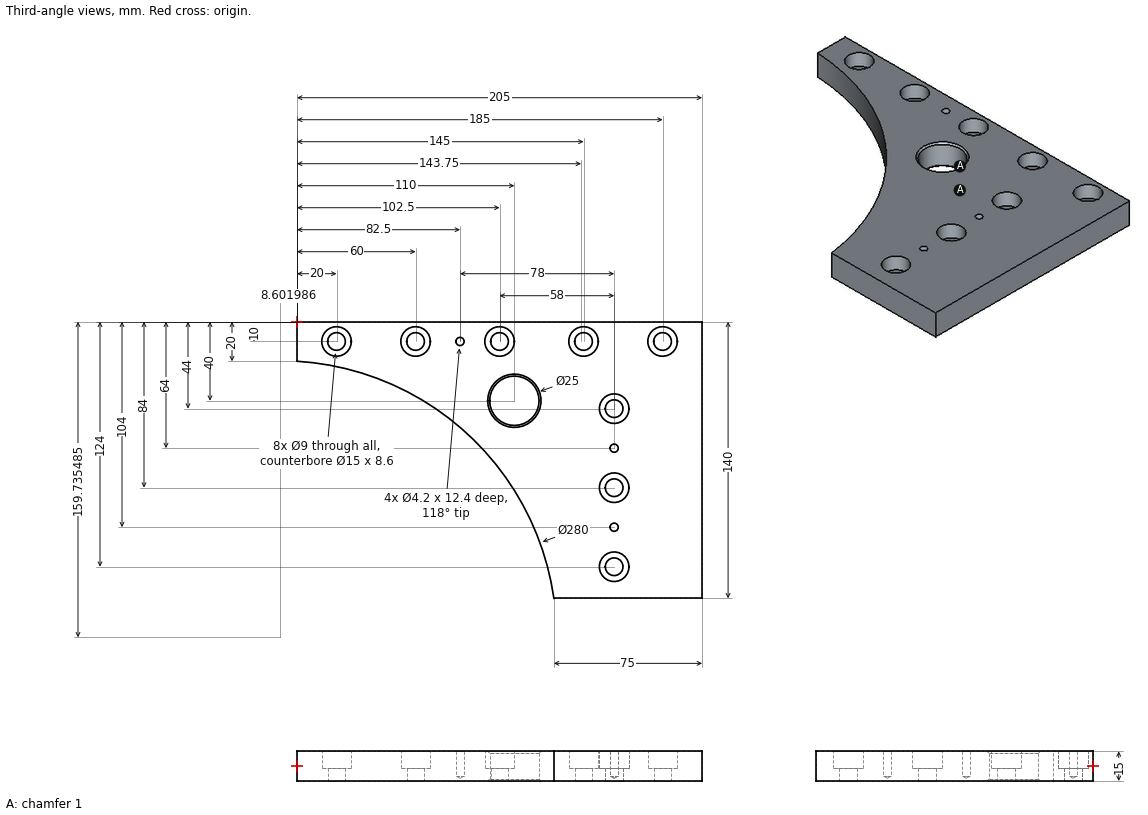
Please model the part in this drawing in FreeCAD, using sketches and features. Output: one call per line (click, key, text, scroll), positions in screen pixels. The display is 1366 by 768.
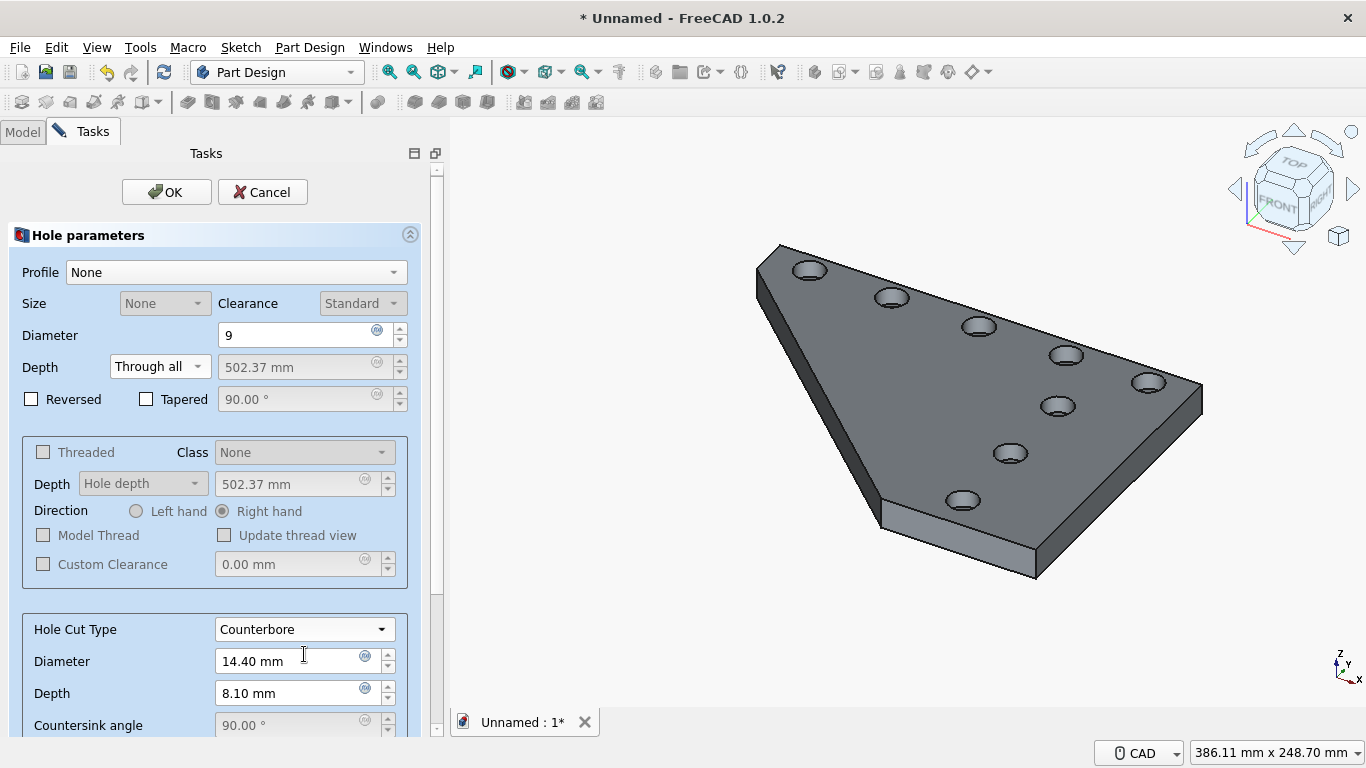
triple_click(298, 661)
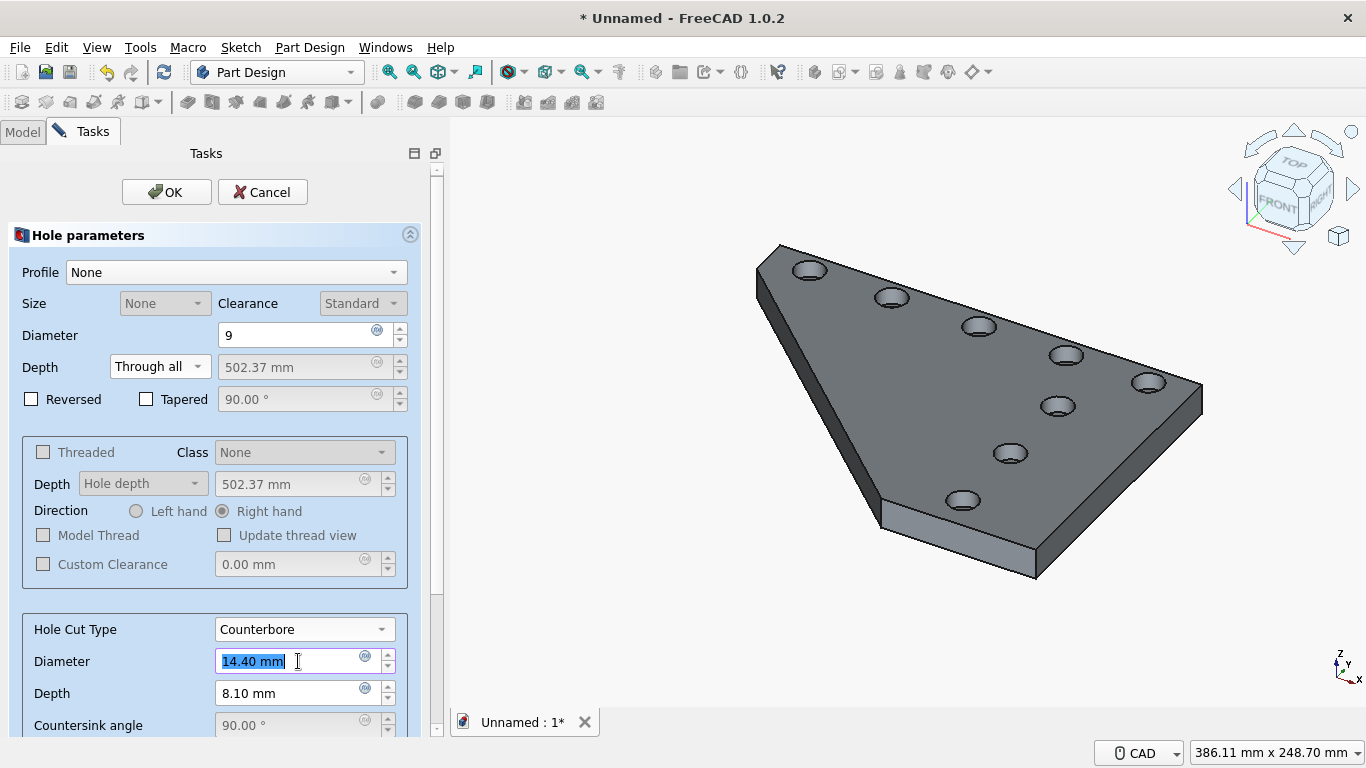
text(15)
key(Tab)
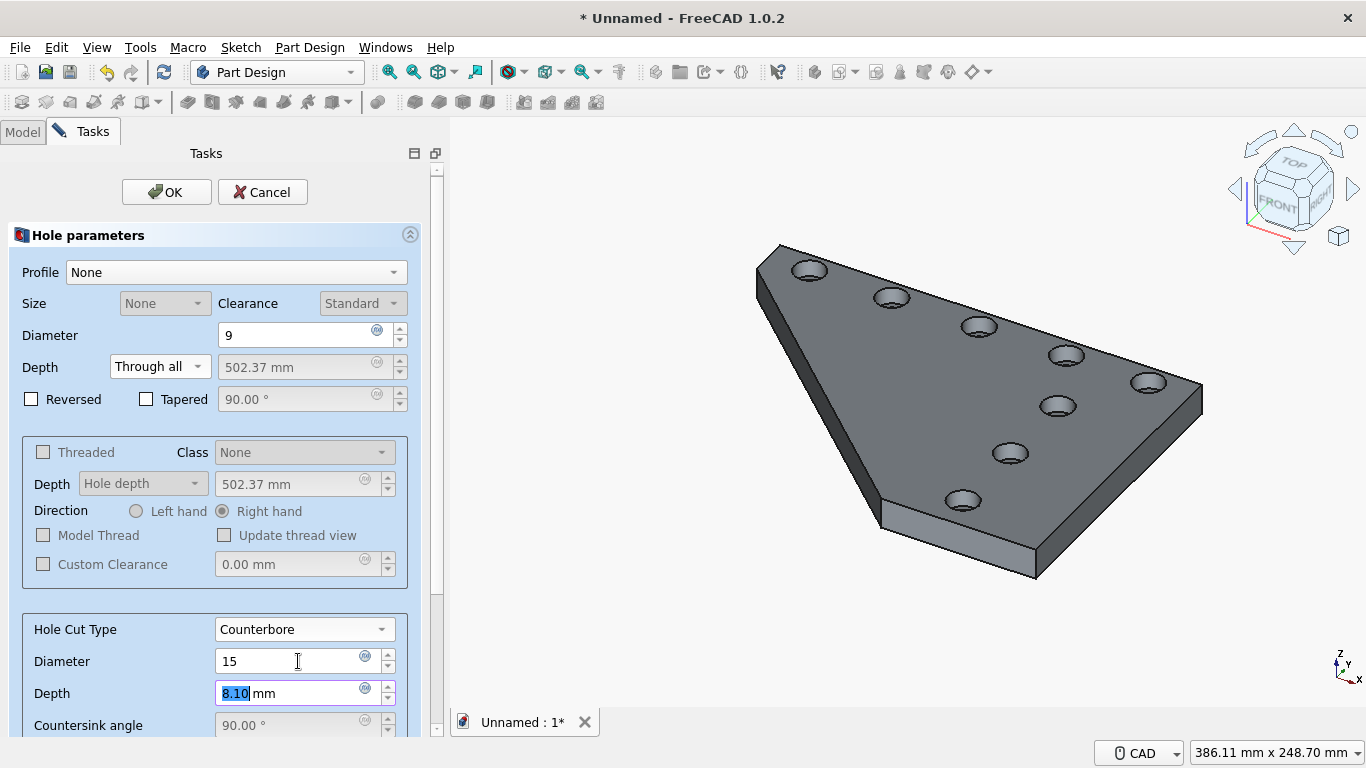
text(8.6)
key(Tab)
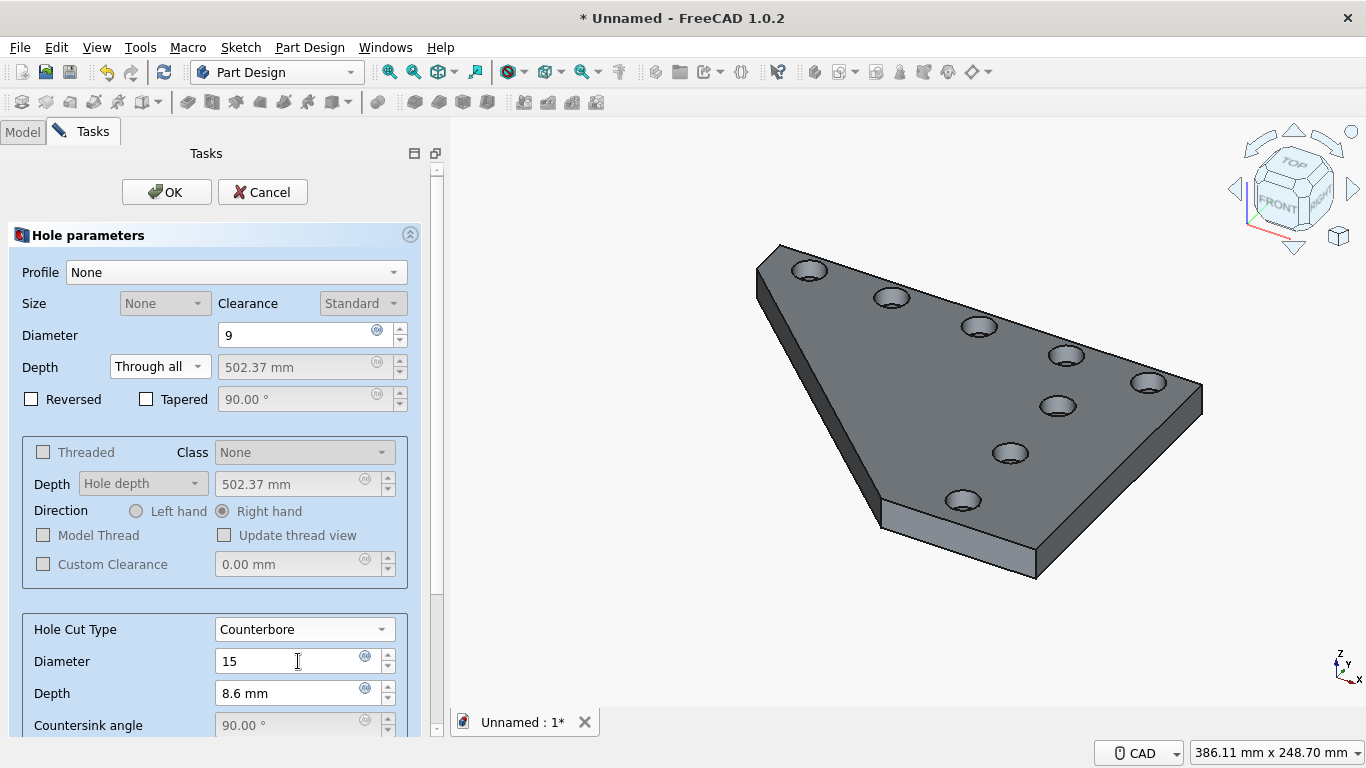
click(167, 192)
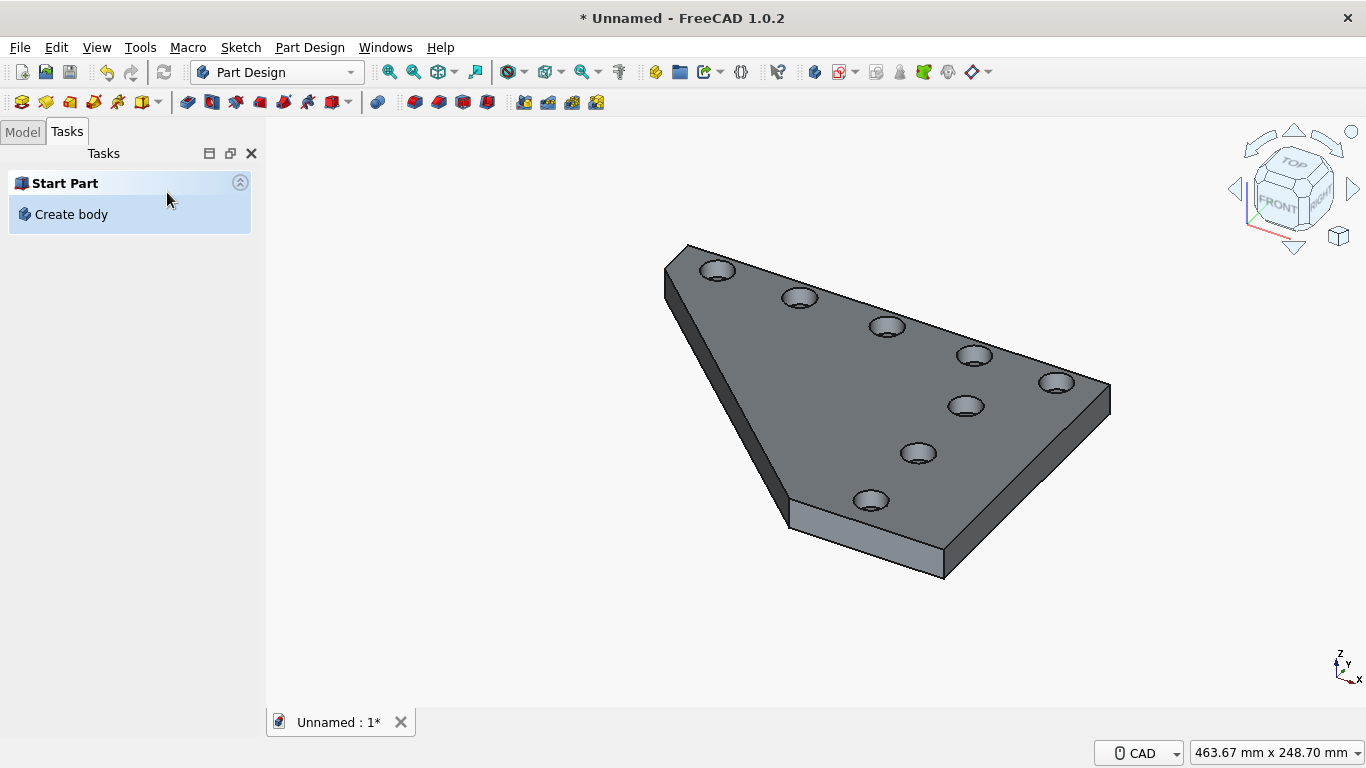
click(816, 396)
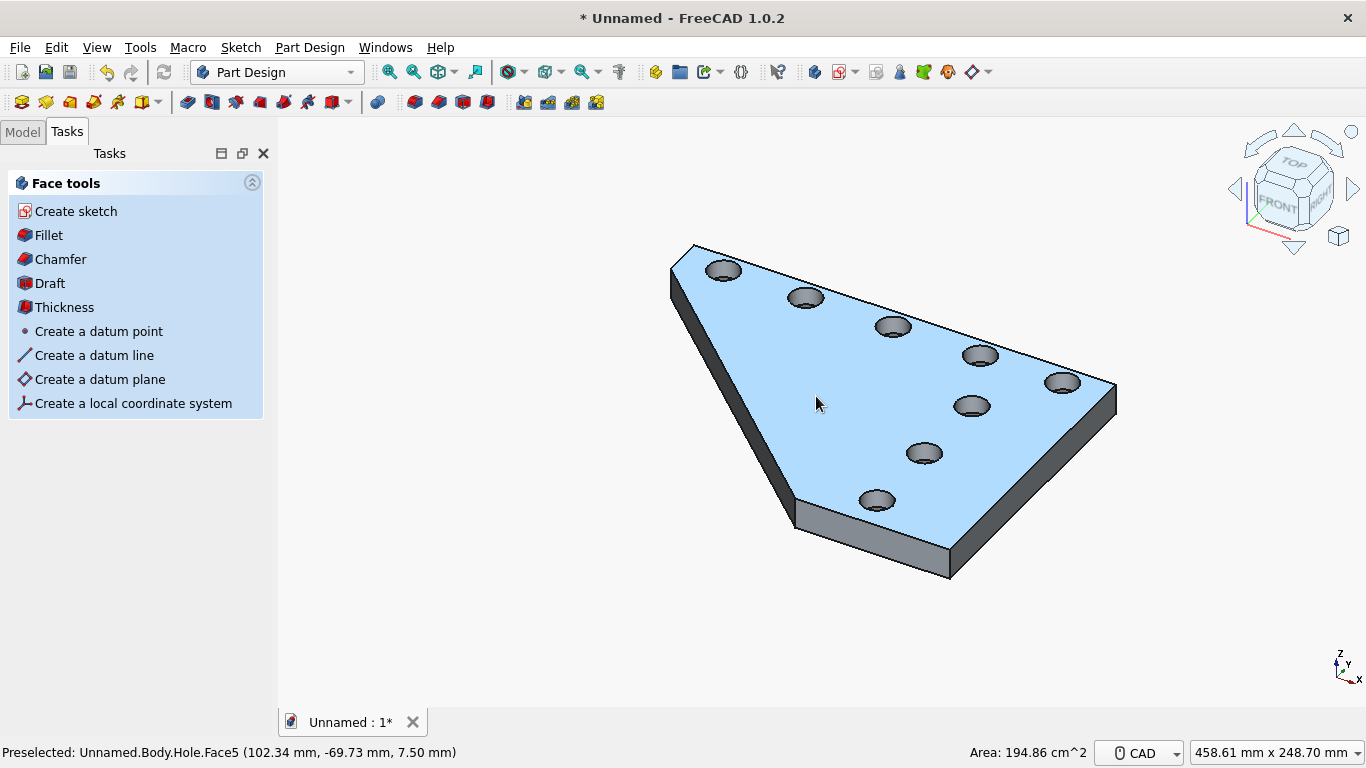
click(840, 72)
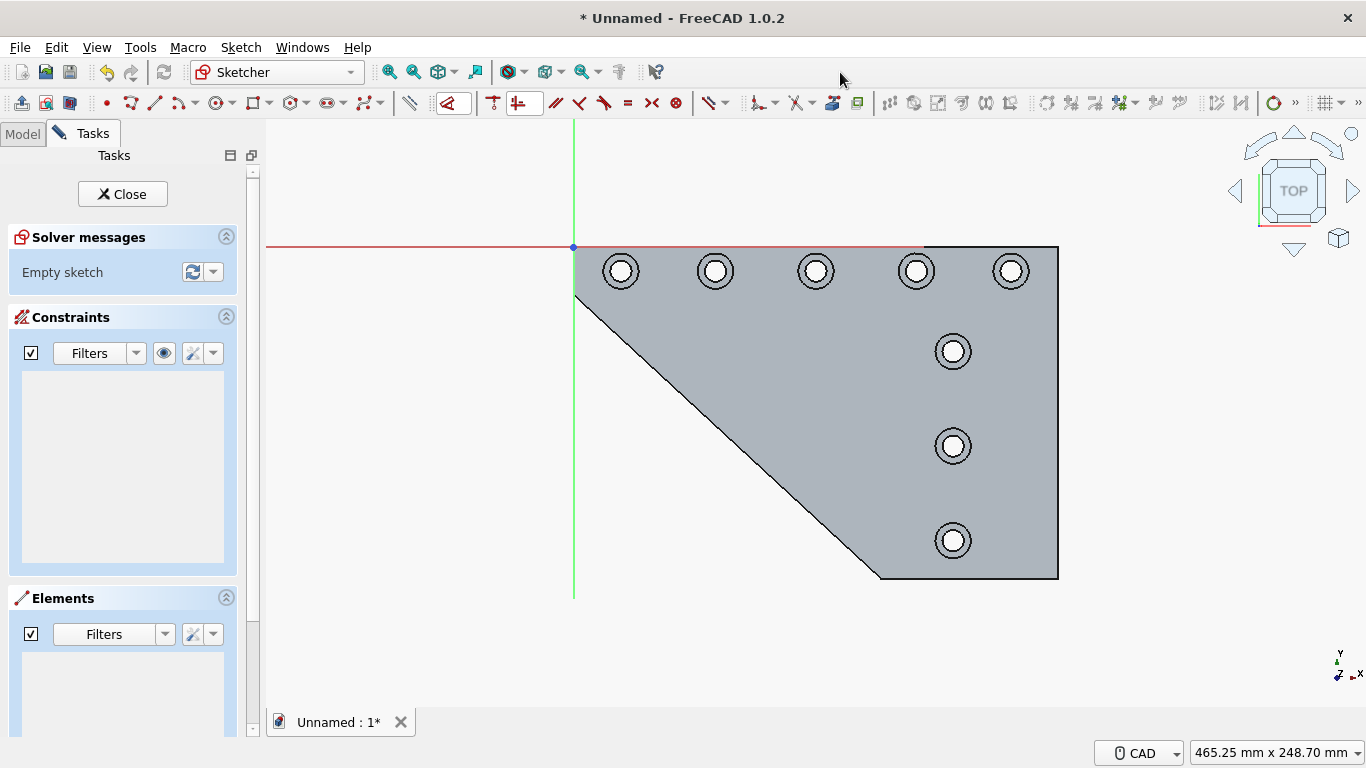
scroll(803, 291, up, 2)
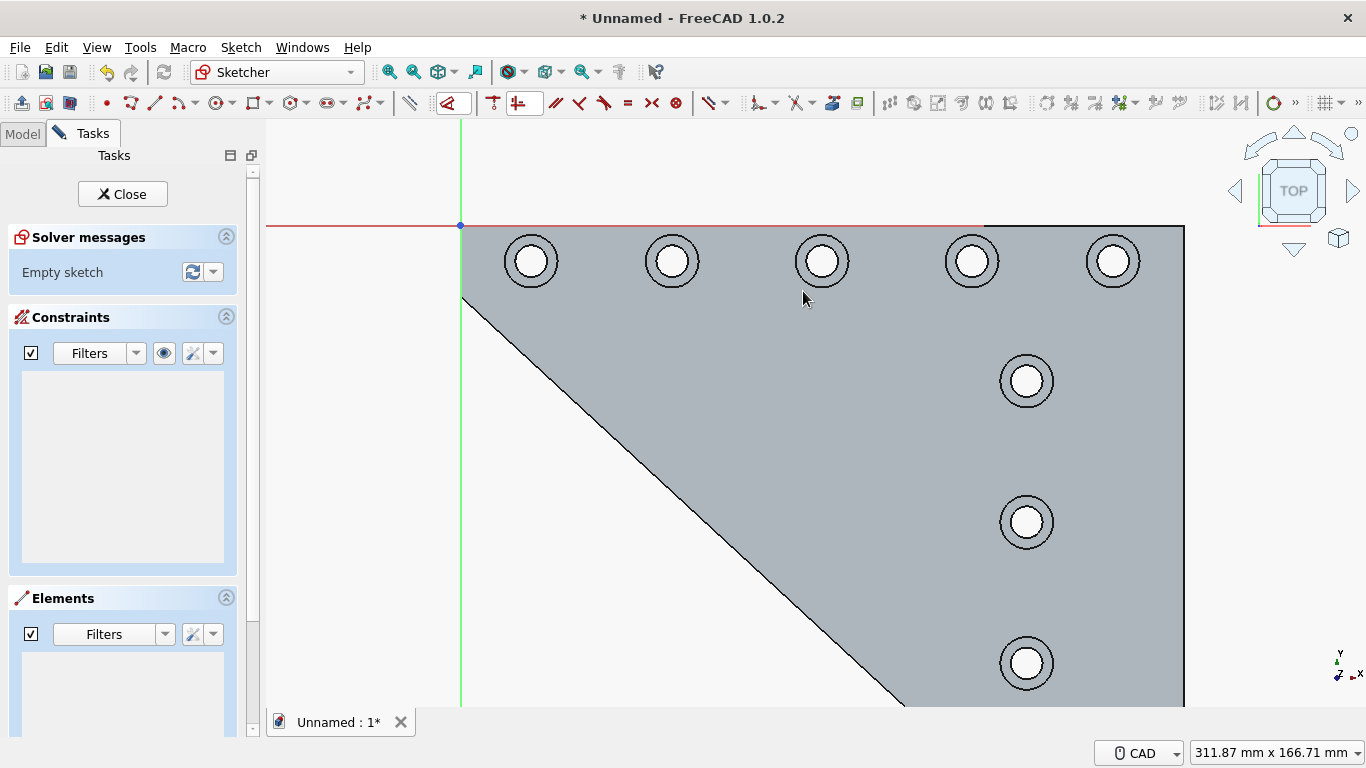
click(216, 104)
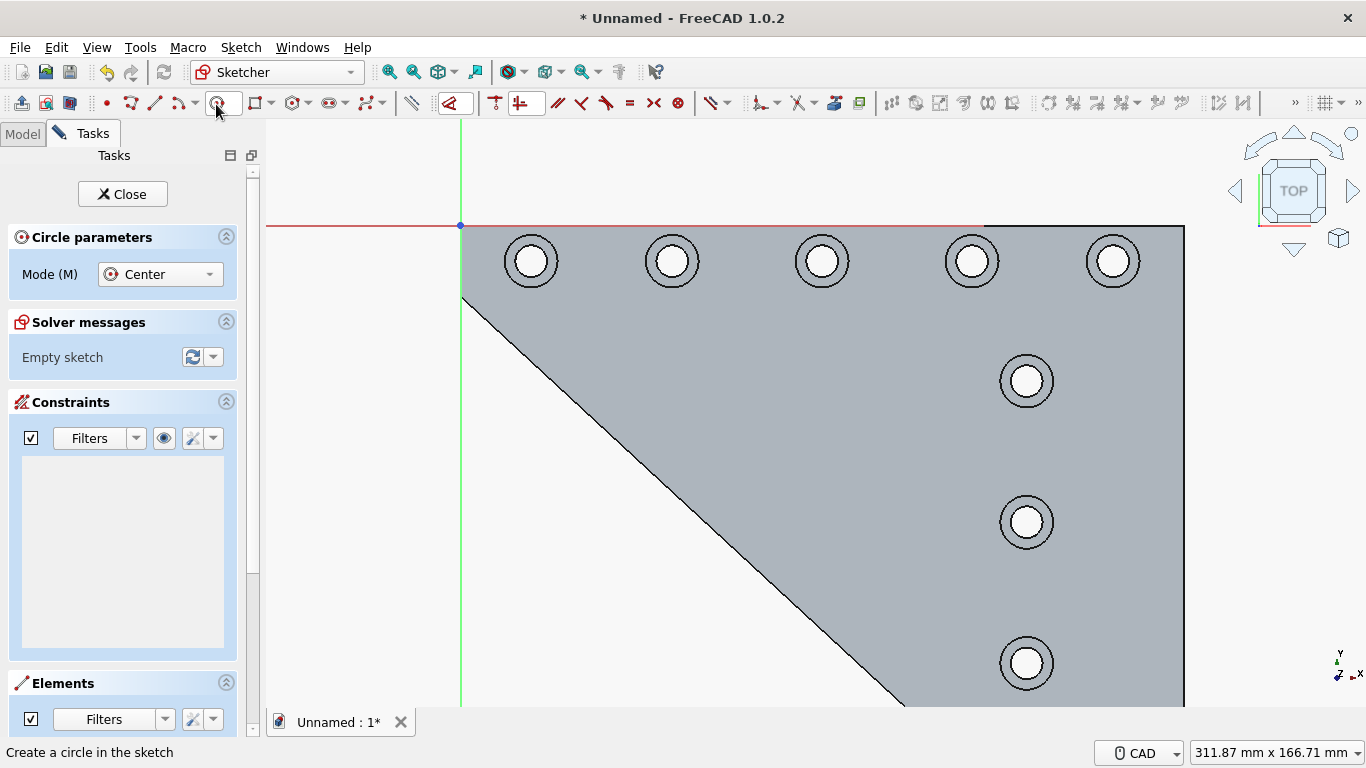
scroll(752, 261, up, 6)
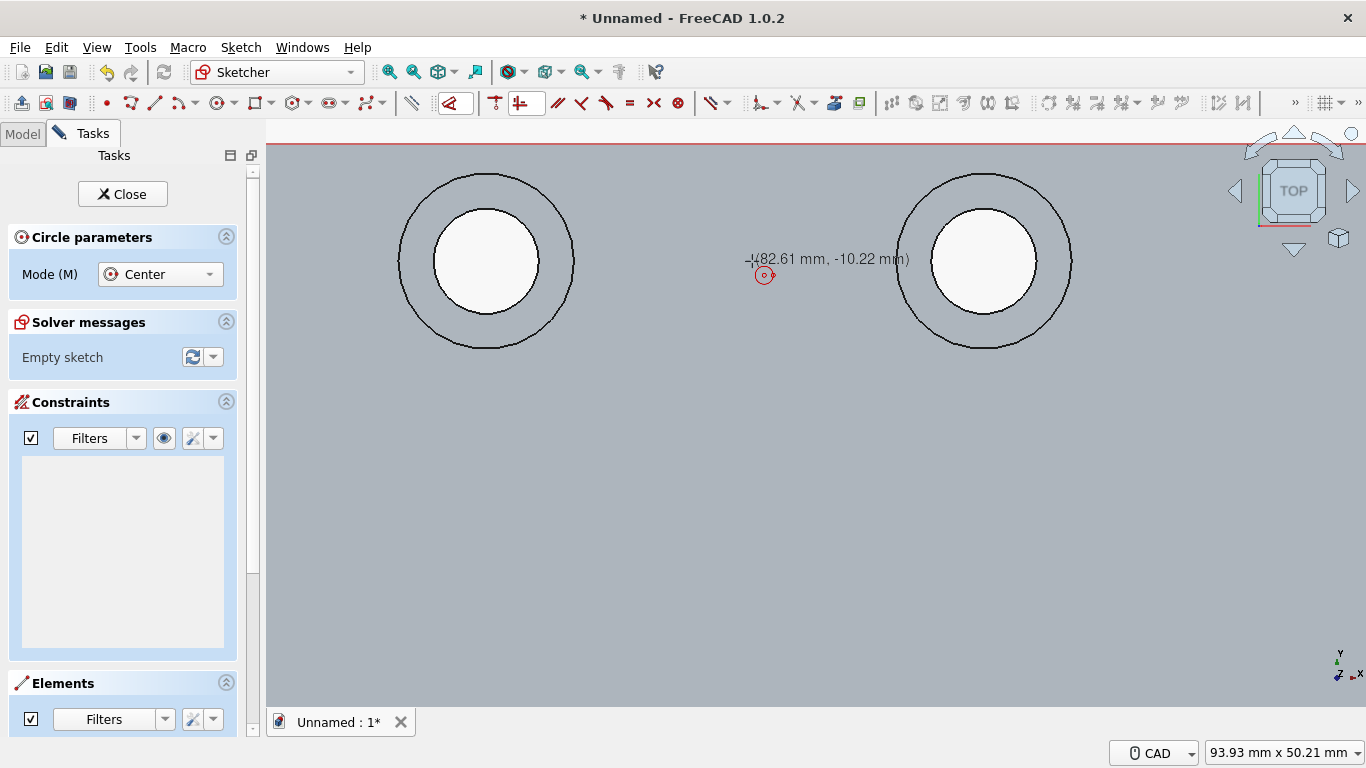
click(750, 261)
click(767, 244)